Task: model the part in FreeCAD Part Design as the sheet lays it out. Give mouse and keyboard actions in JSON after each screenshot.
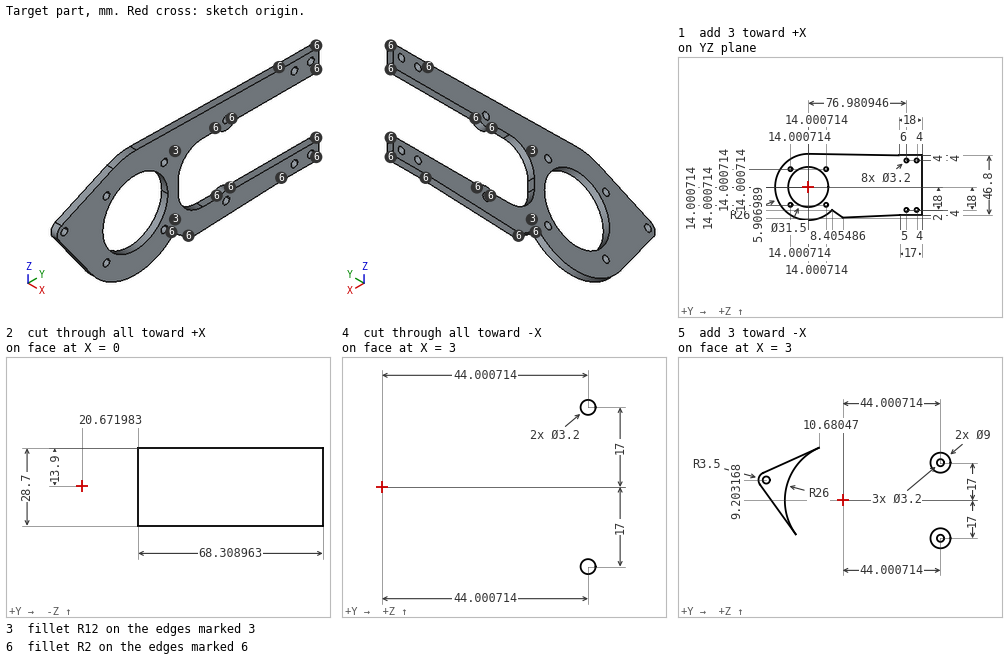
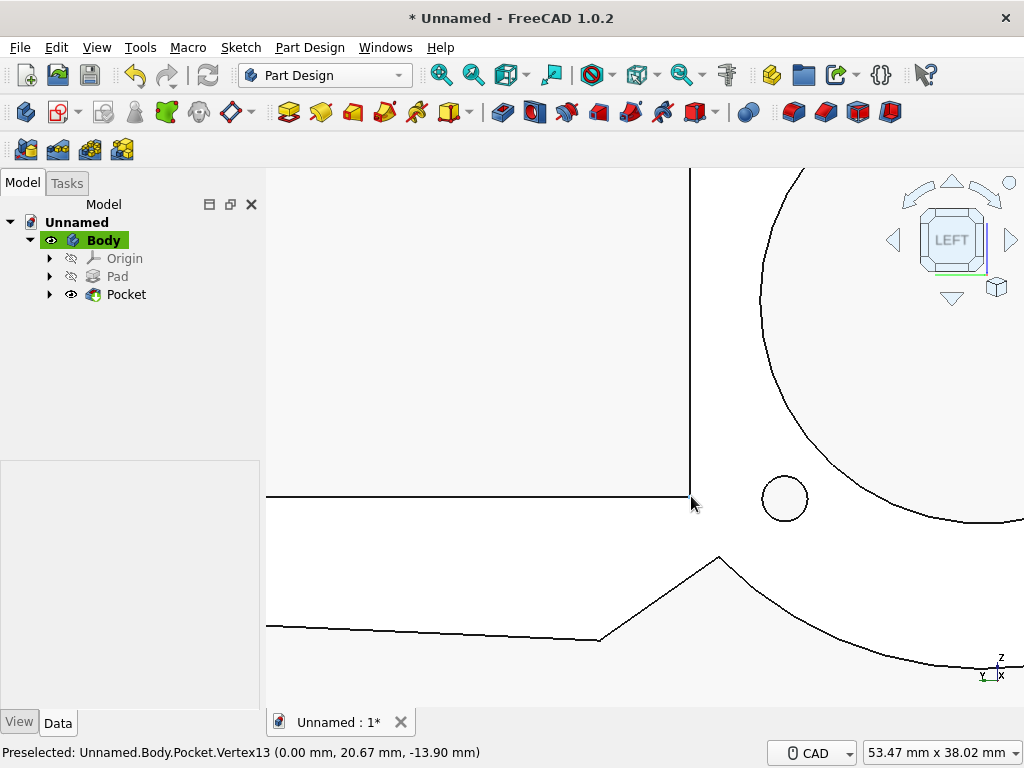
{"action": "left_click", "coordinate": [442, 76]}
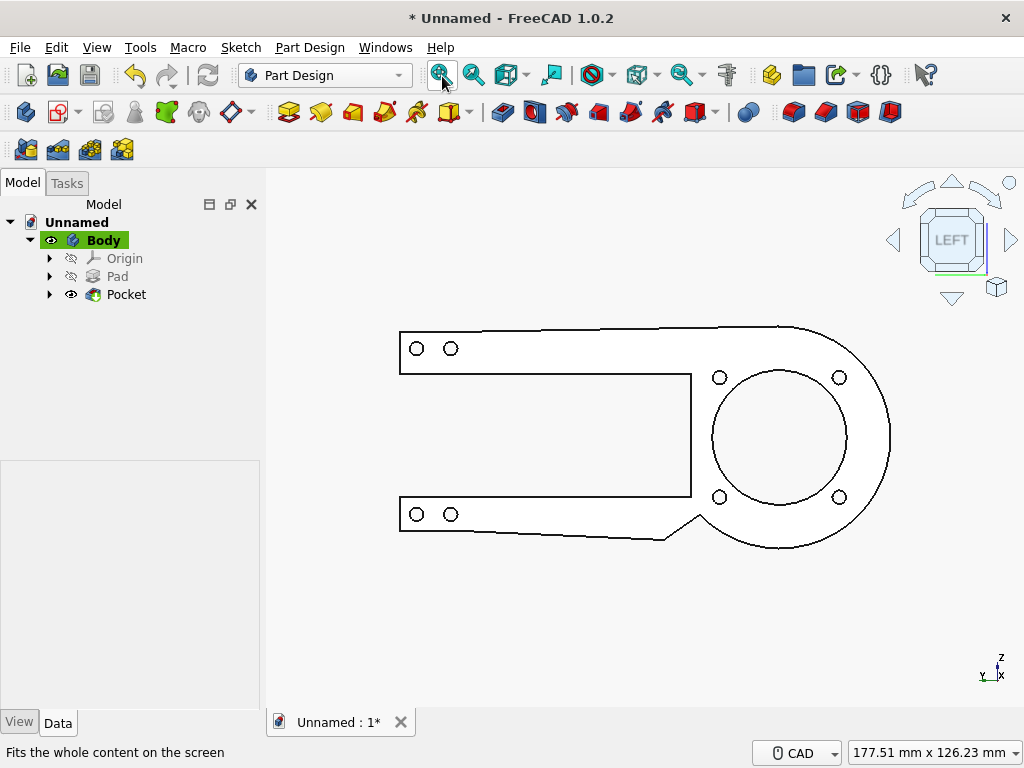
{"action": "key", "text": "0"}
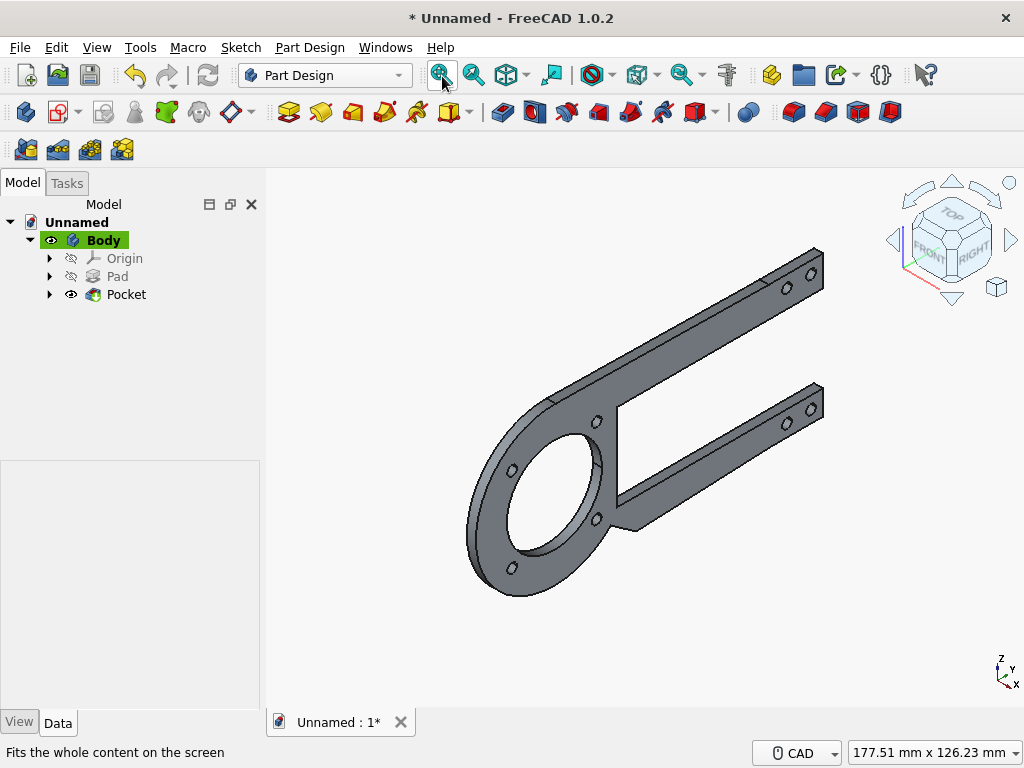
{"action": "scroll", "coordinate": [612, 504], "scroll_direction": "up", "scroll_amount": 6}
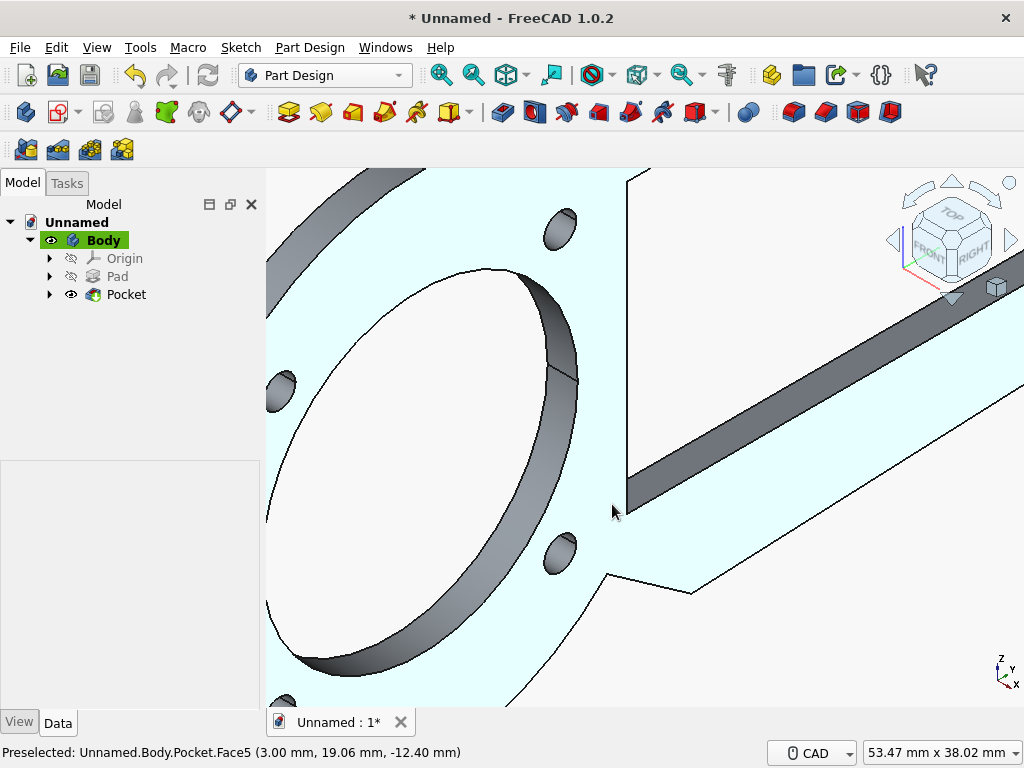
{"action": "left_click", "coordinate": [442, 76]}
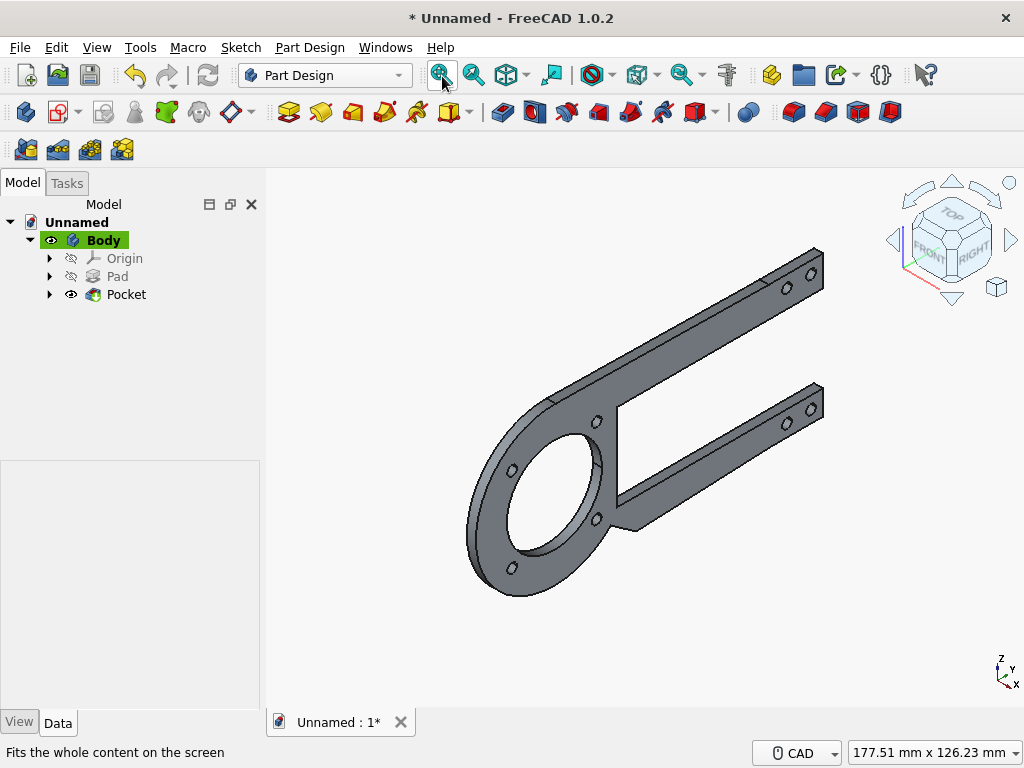
{"action": "key", "text": "2"}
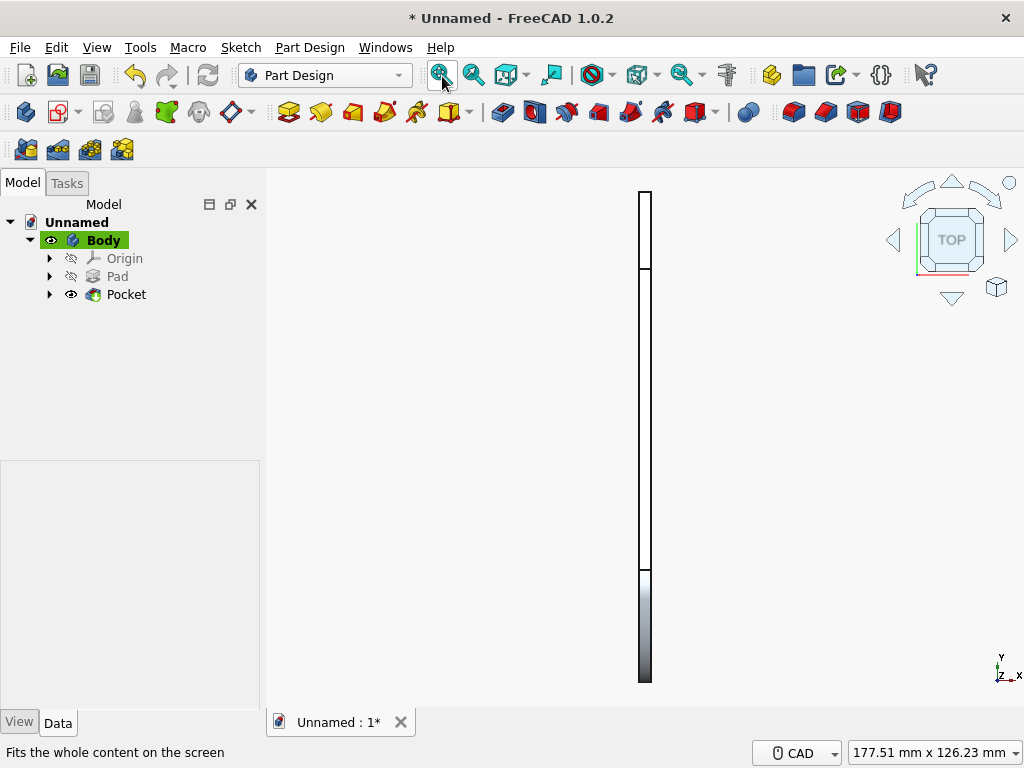
{"action": "scroll", "coordinate": [645, 483], "scroll_direction": "up", "scroll_amount": 6}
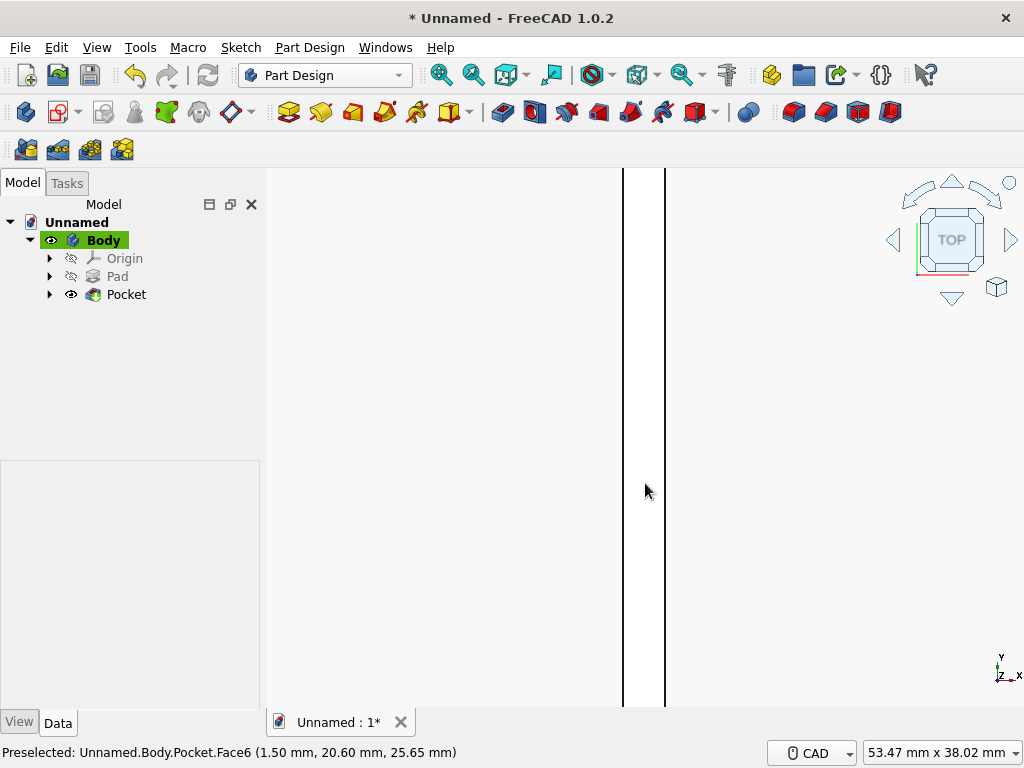
{"action": "left_click", "coordinate": [442, 76]}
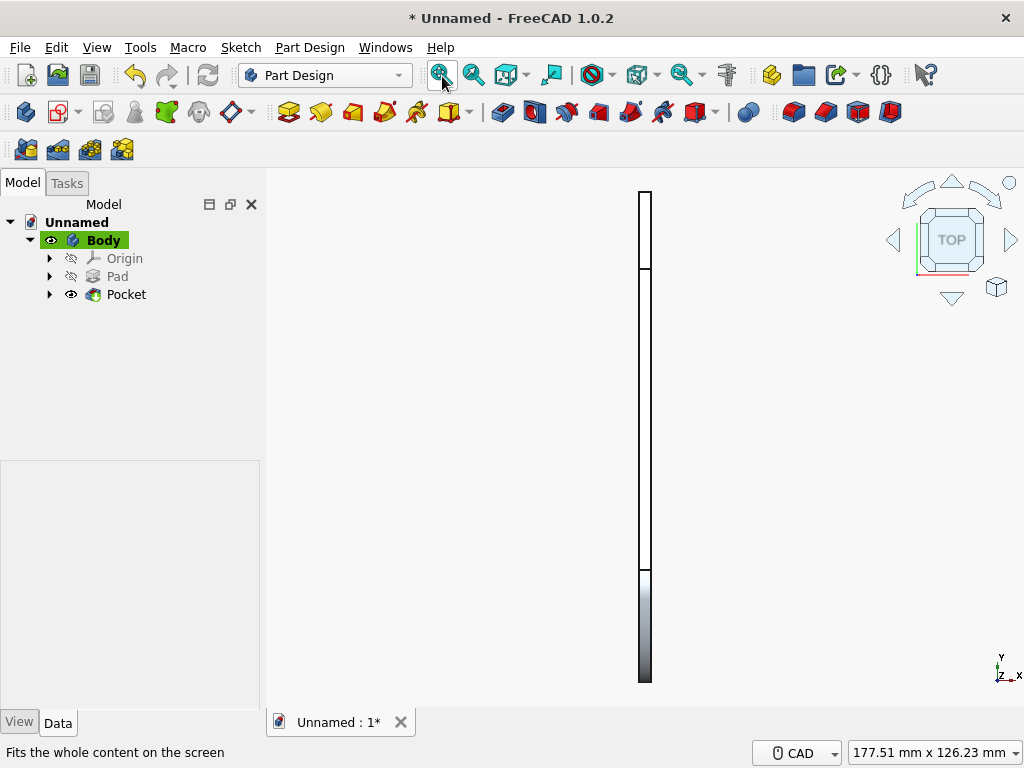
{"action": "key", "text": "1"}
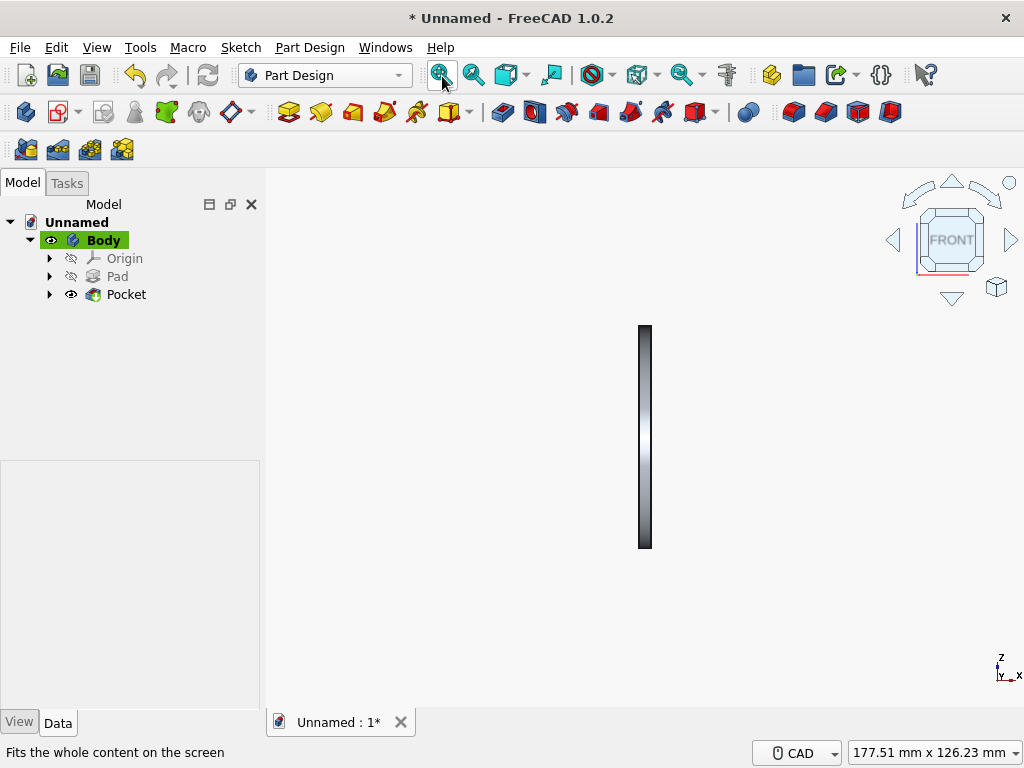
{"action": "left_click", "coordinate": [442, 76]}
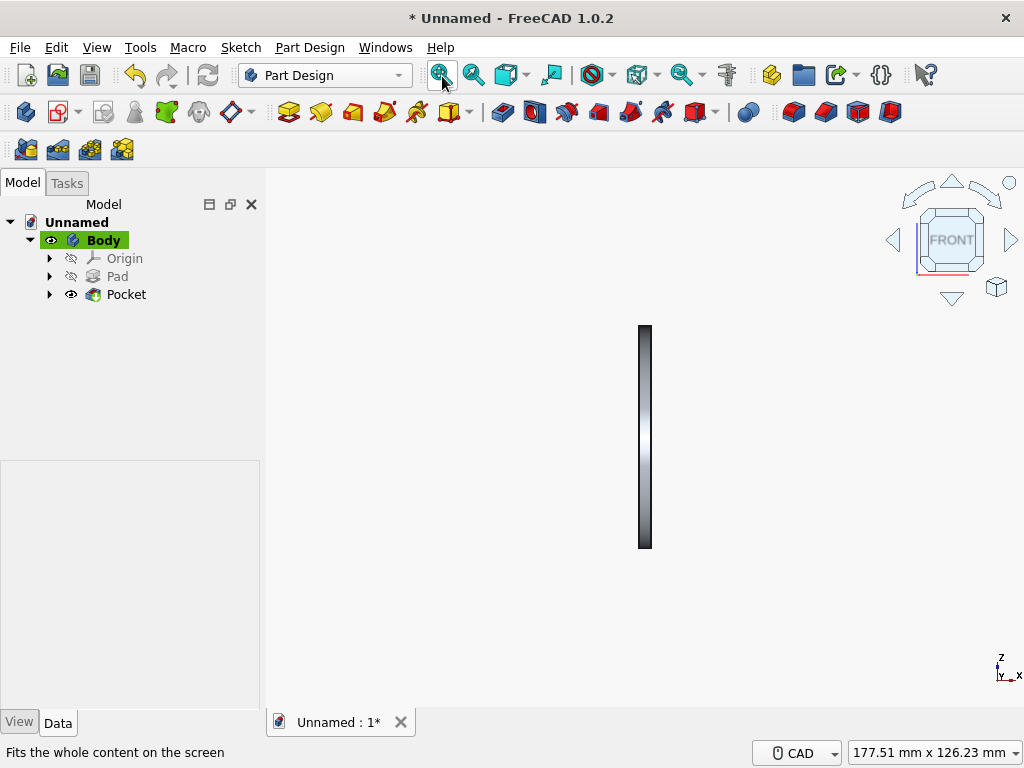
{"action": "scroll", "coordinate": [645, 496], "scroll_direction": "up", "scroll_amount": 6}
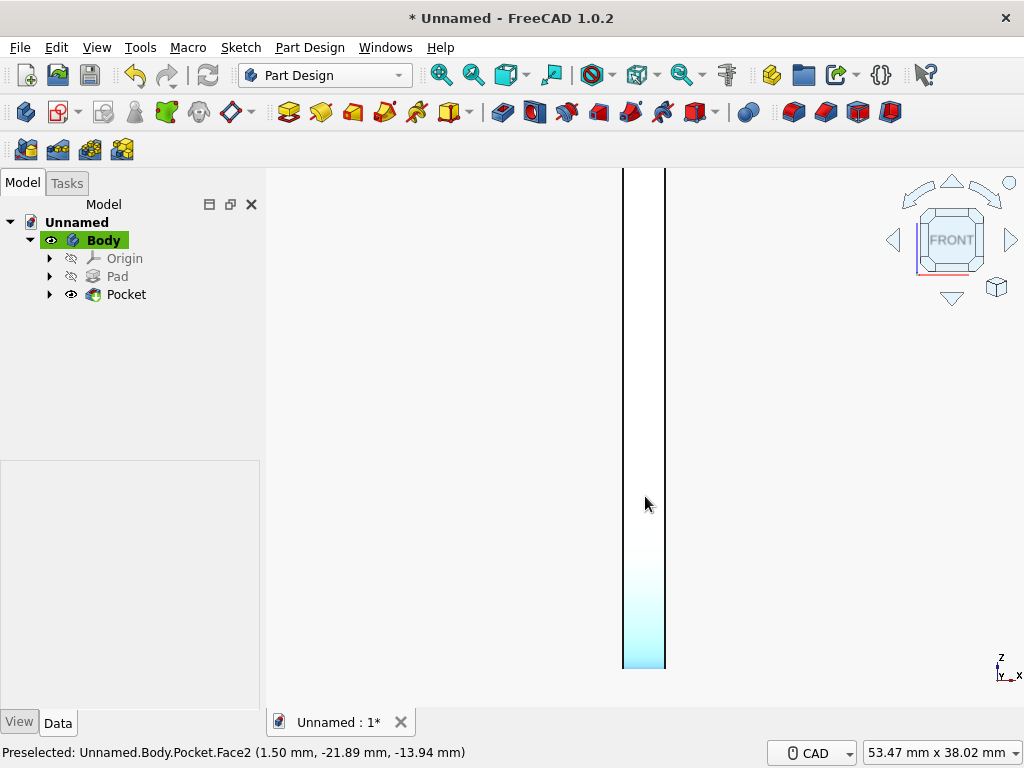
{"action": "left_click", "coordinate": [442, 76]}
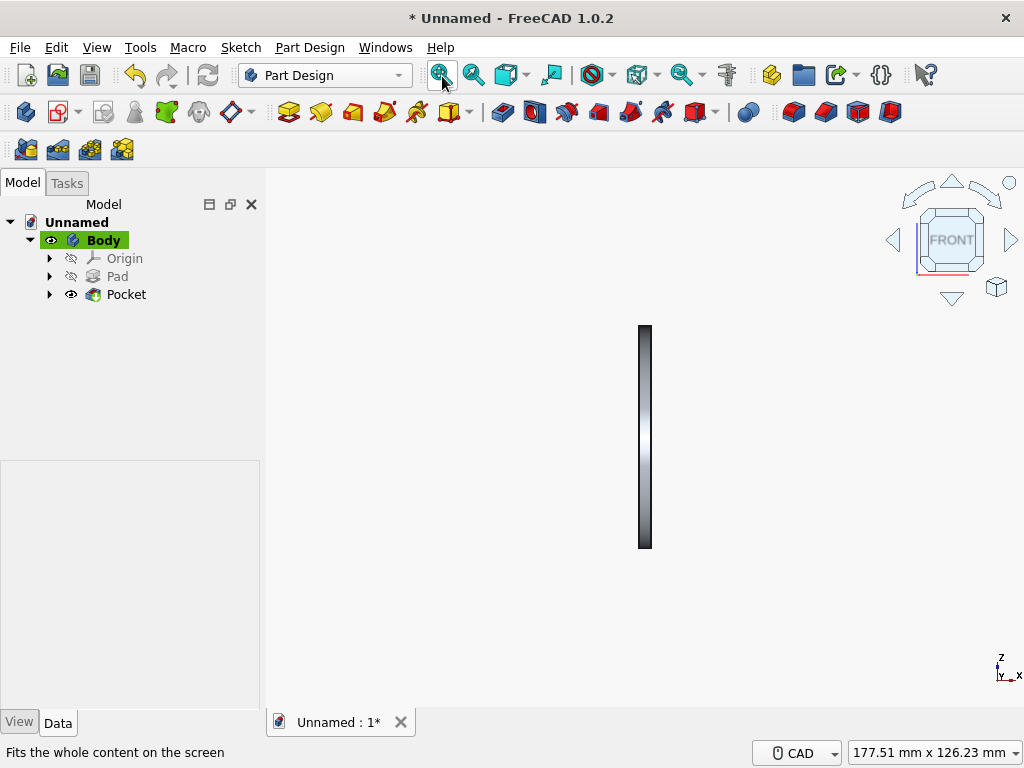
{"action": "key", "text": "3"}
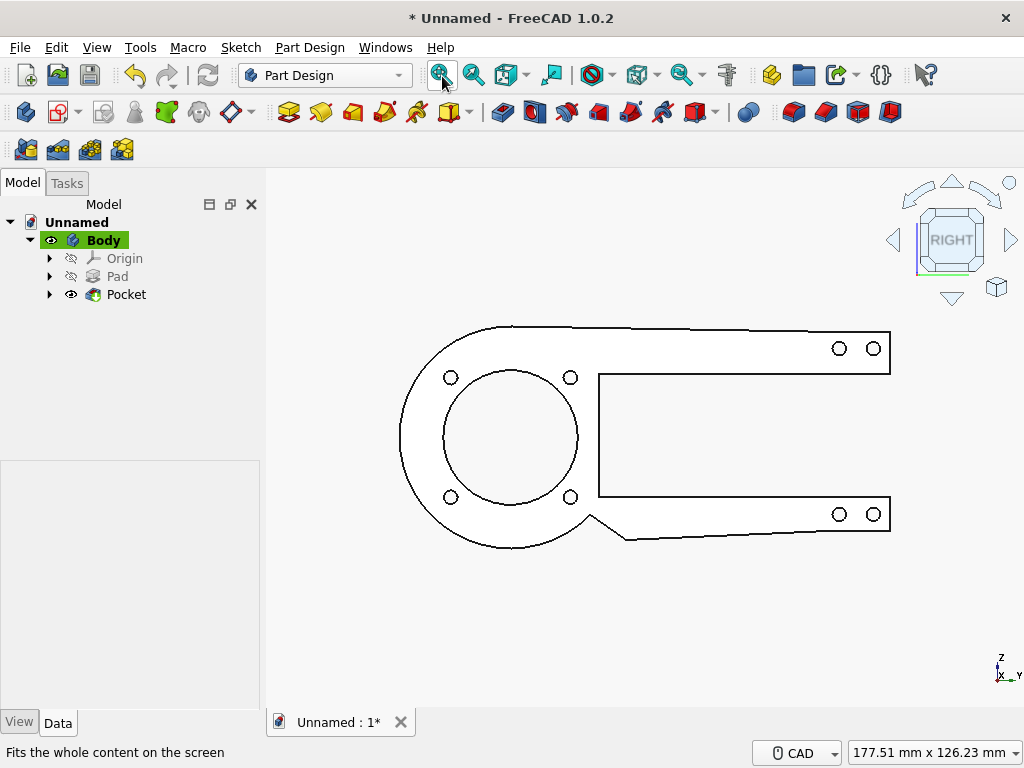
{"action": "scroll", "coordinate": [599, 496], "scroll_direction": "up", "scroll_amount": 6}